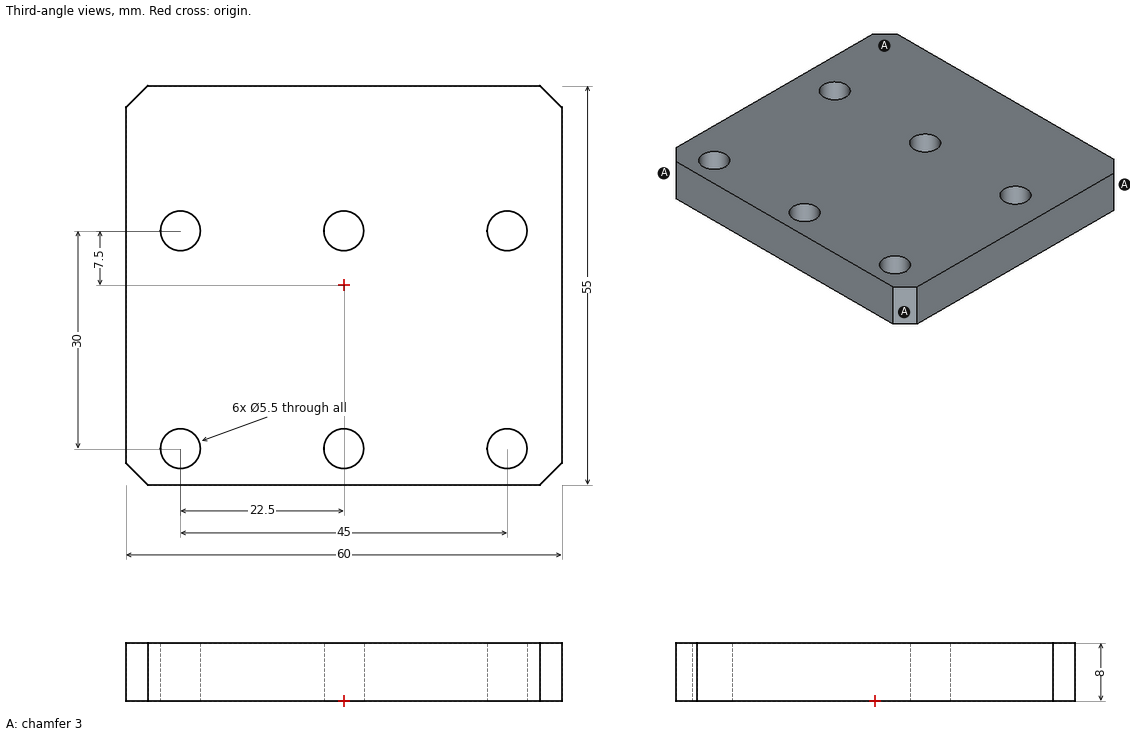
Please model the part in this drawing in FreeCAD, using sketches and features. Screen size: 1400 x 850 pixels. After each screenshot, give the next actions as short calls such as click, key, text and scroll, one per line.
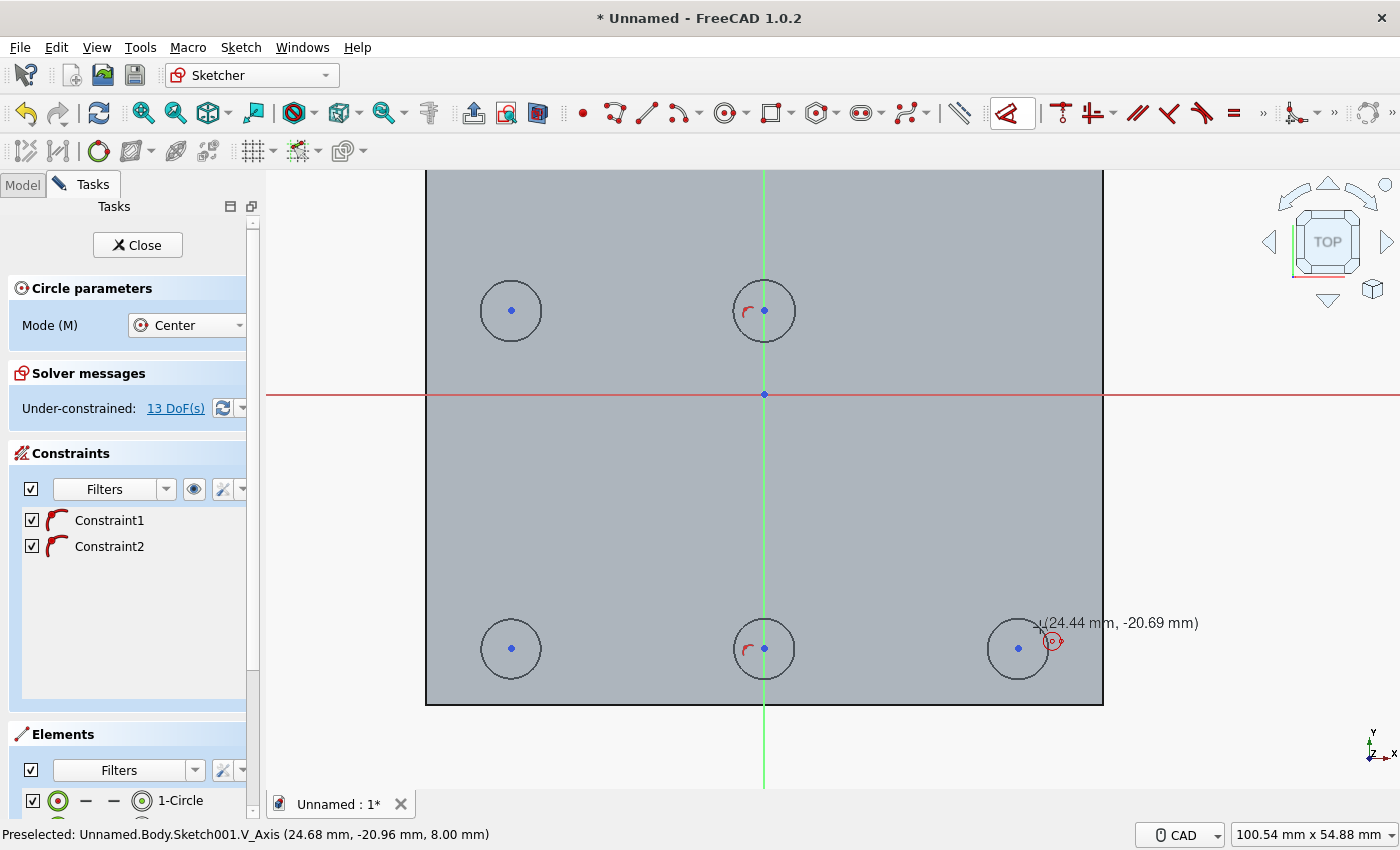
click(1018, 310)
click(1040, 288)
key(Escape)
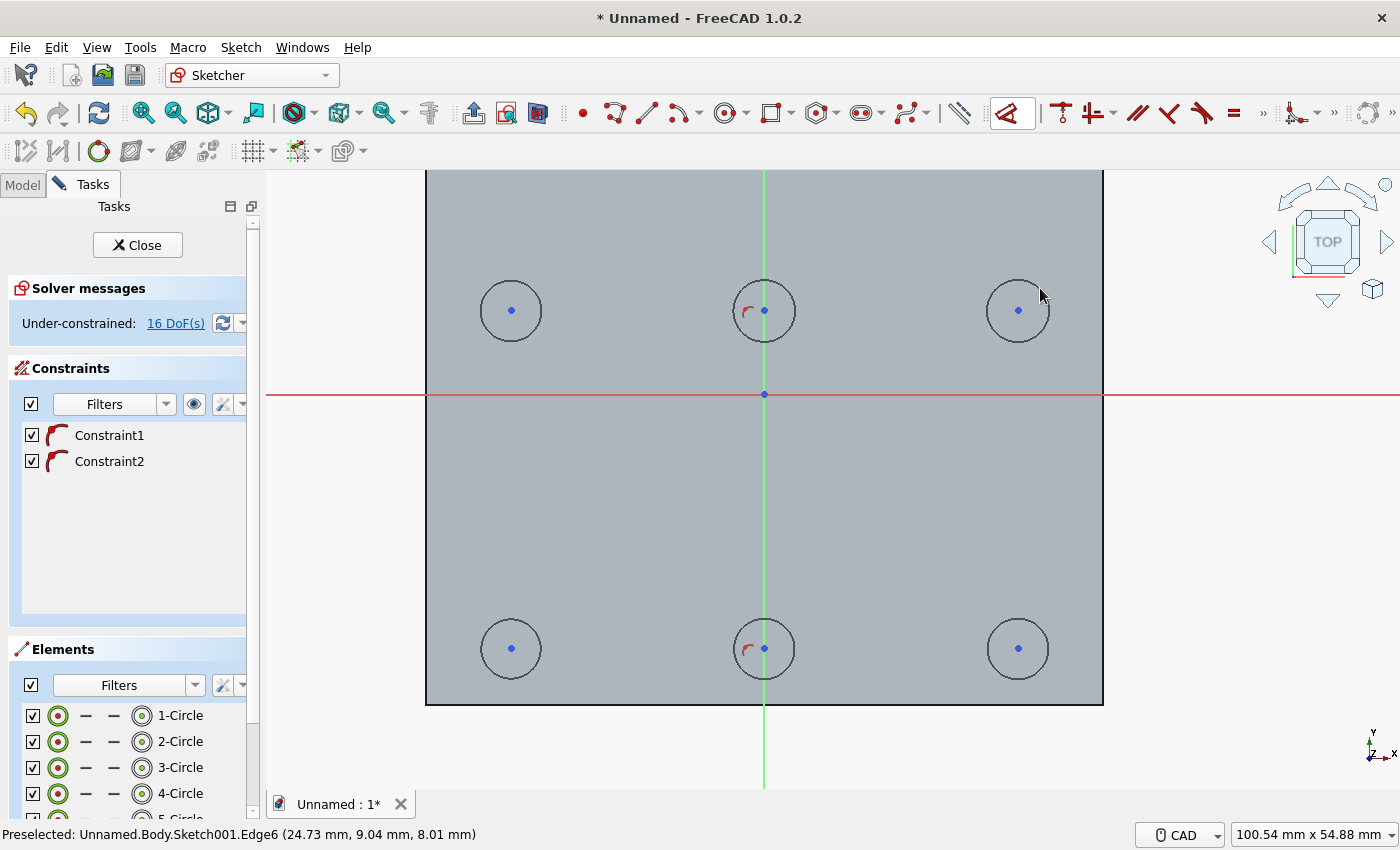
click(532, 628)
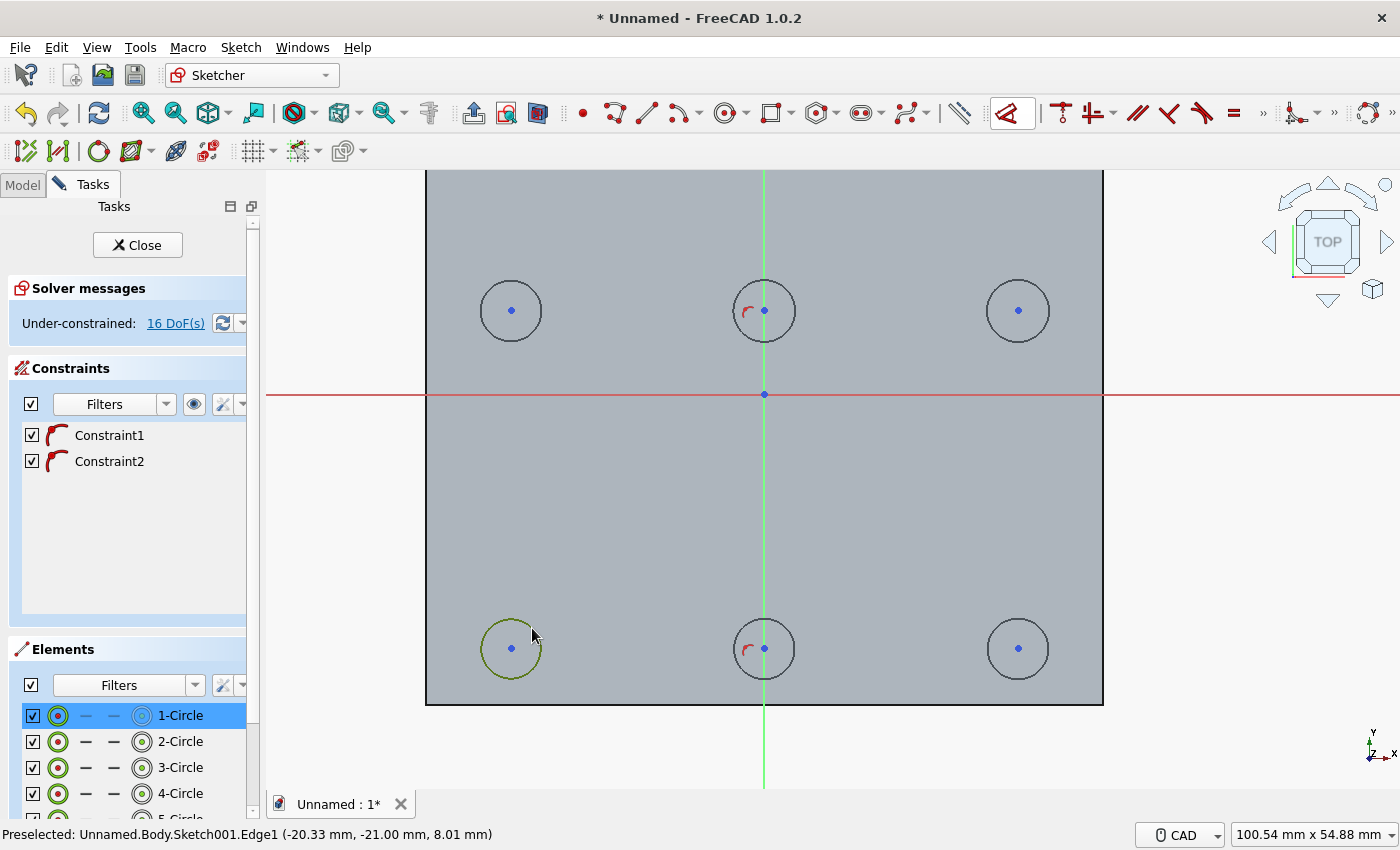
click(532, 289)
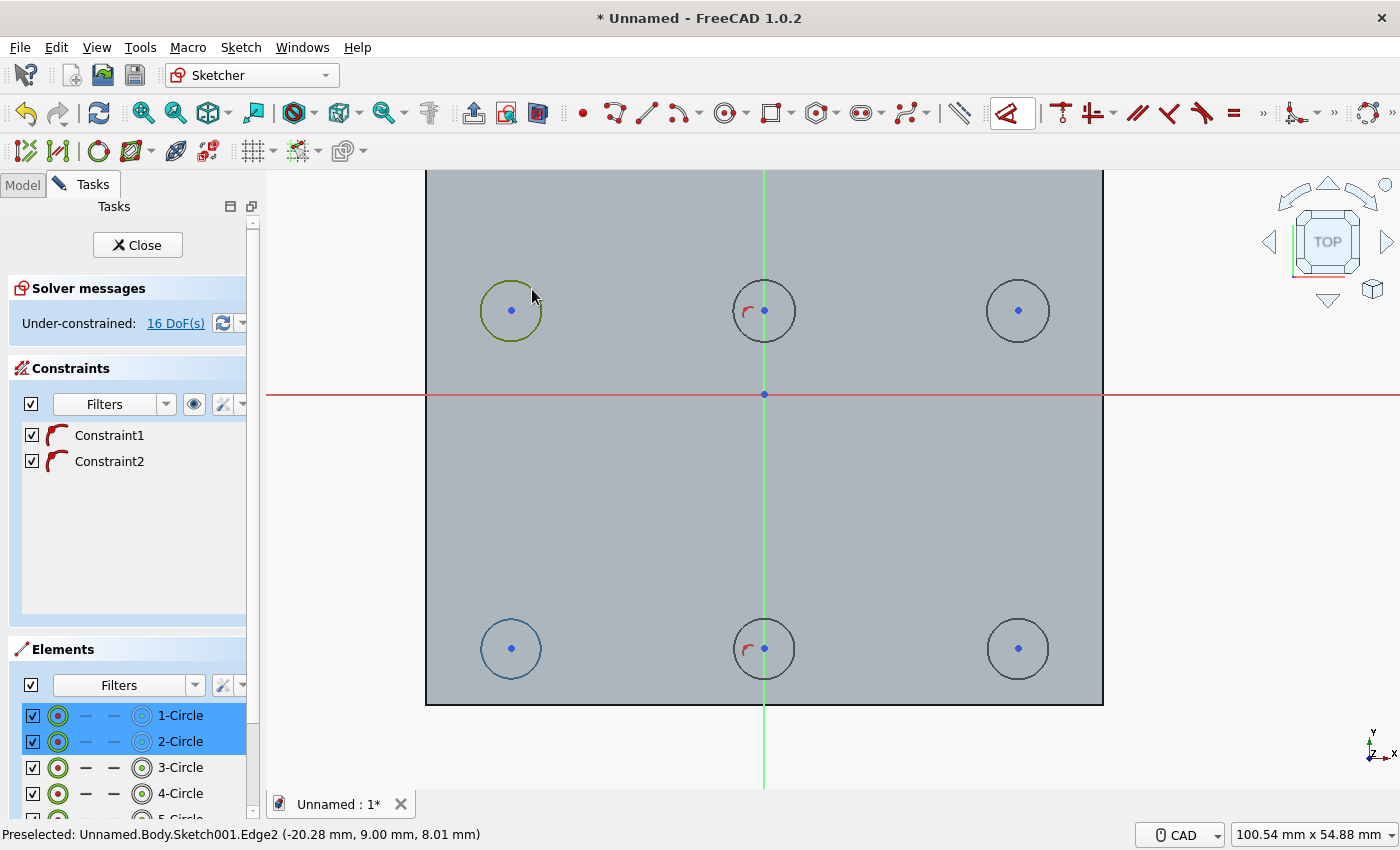
click(786, 289)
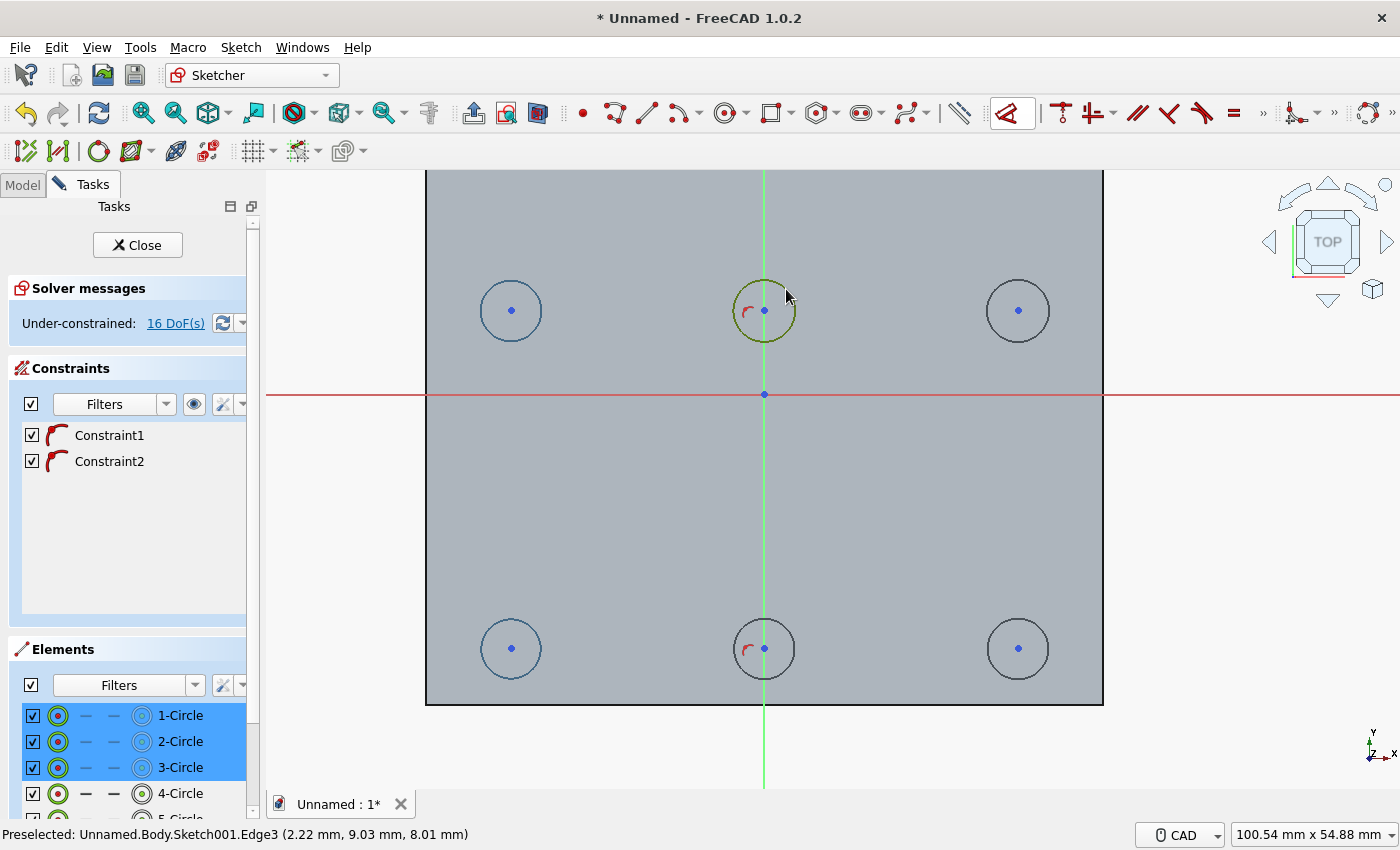
click(786, 628)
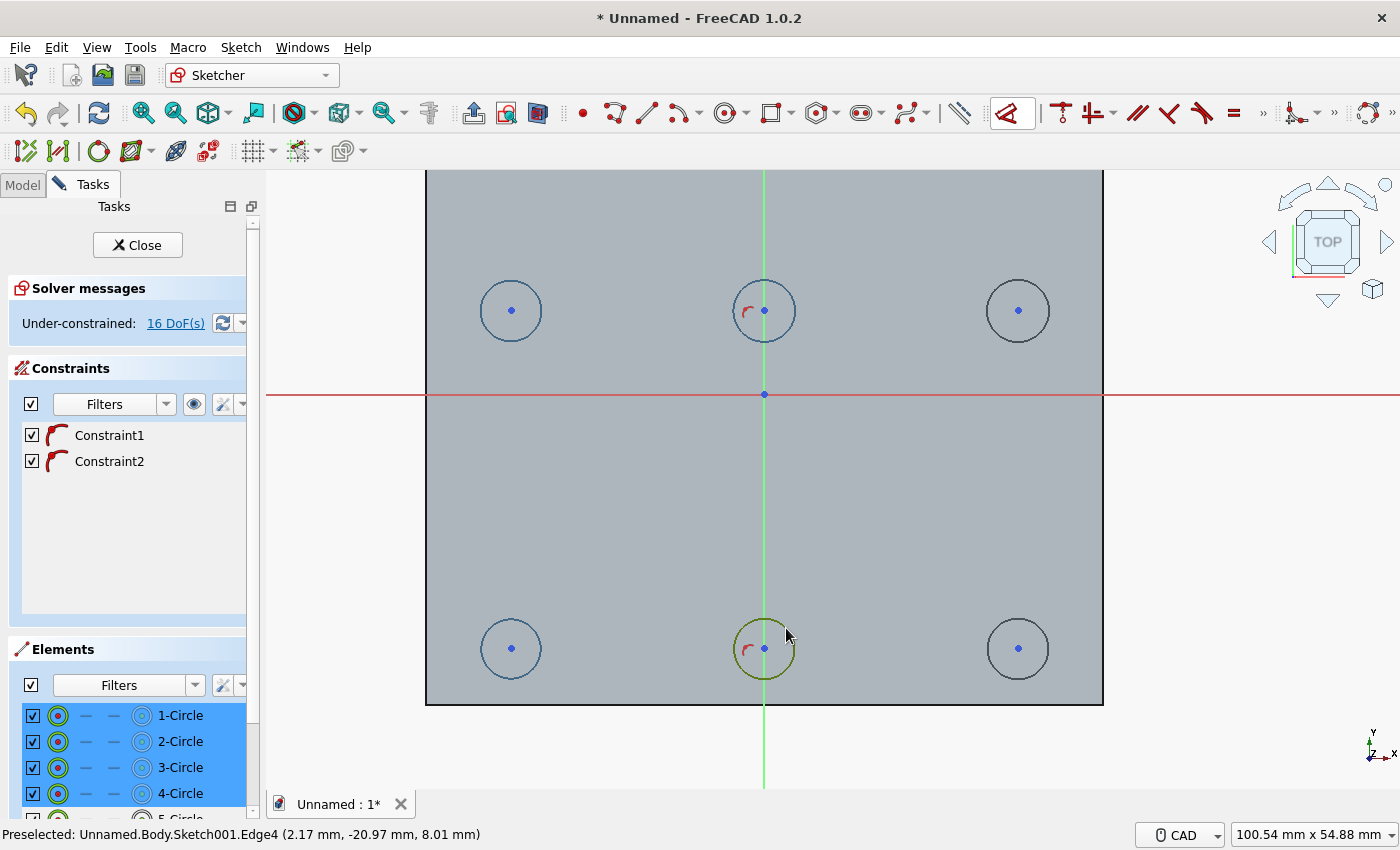
click(1039, 627)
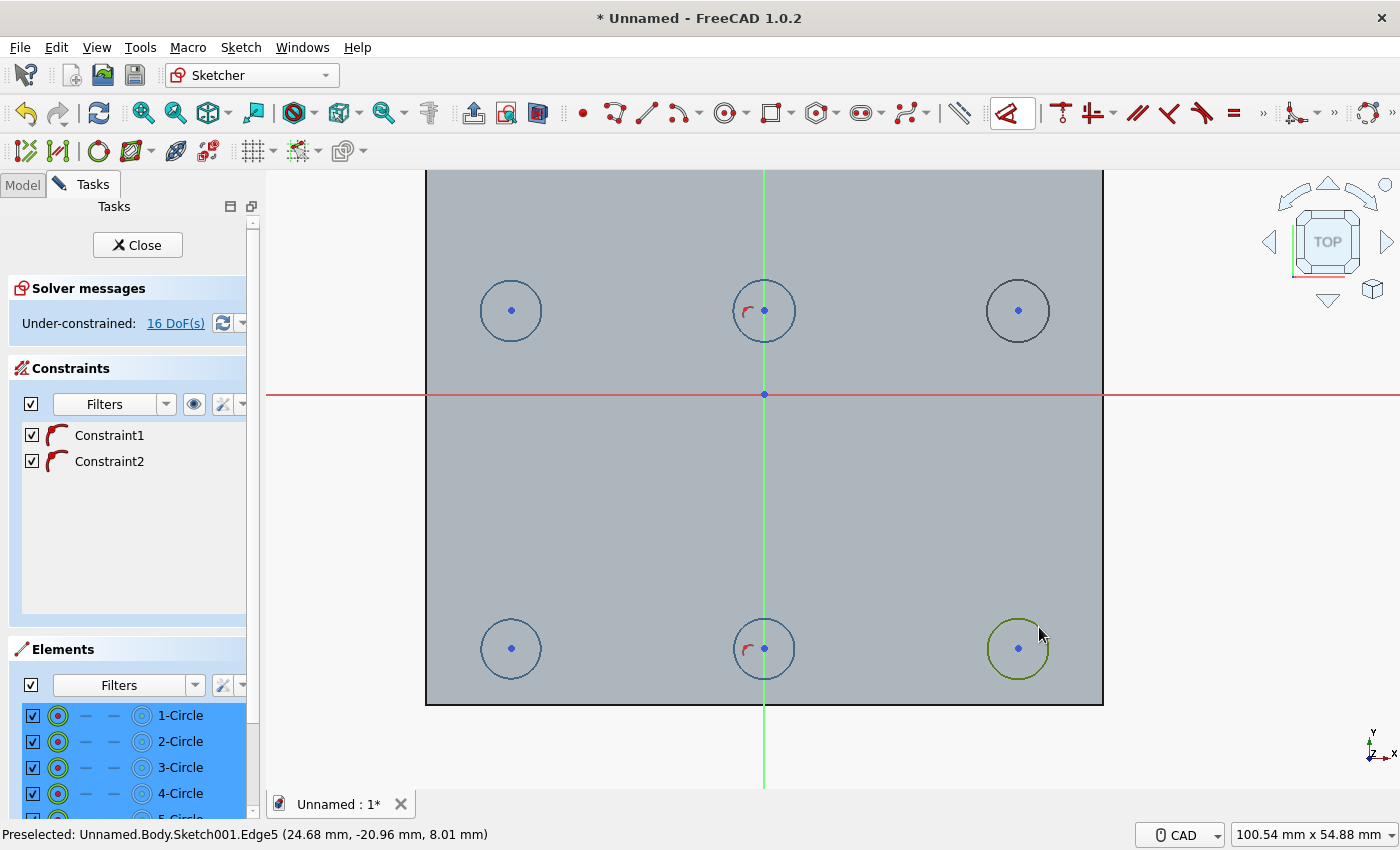
click(1040, 289)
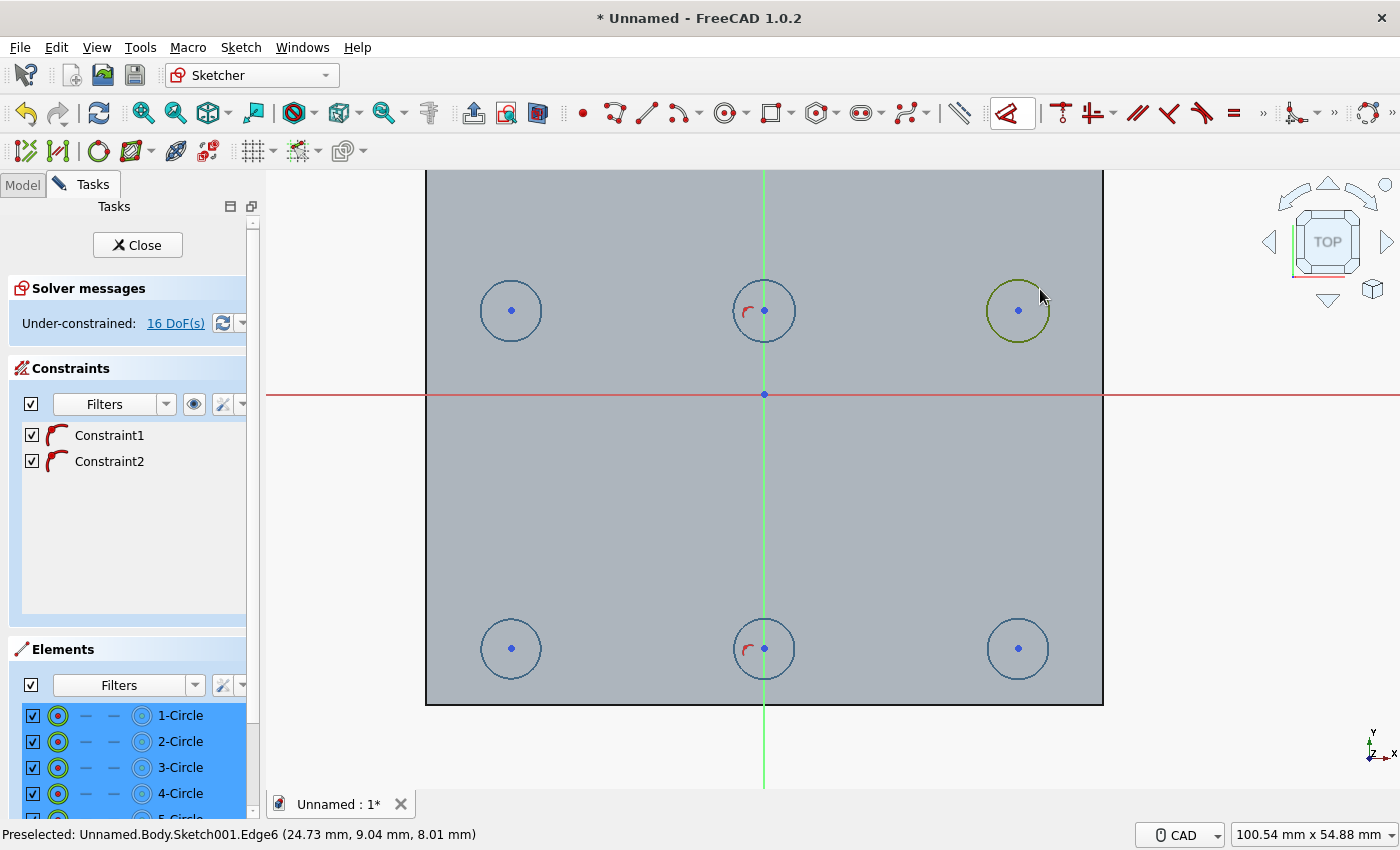
click(1234, 114)